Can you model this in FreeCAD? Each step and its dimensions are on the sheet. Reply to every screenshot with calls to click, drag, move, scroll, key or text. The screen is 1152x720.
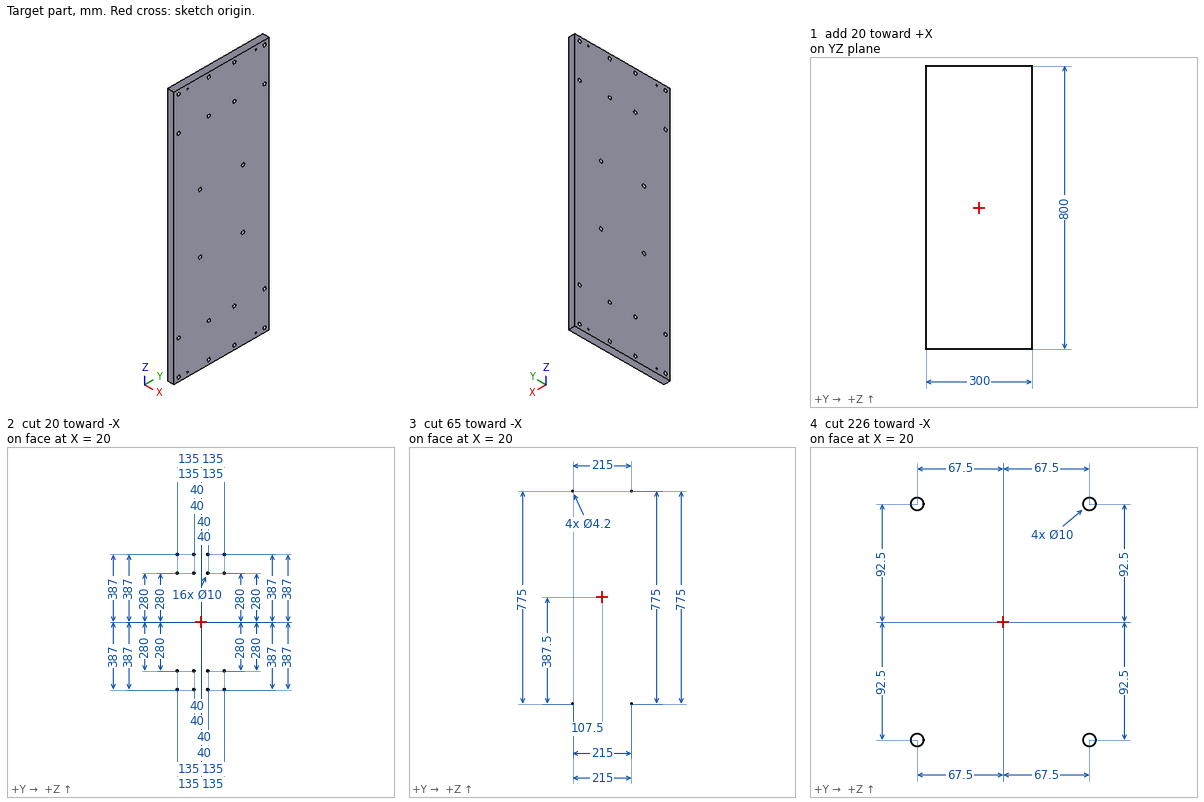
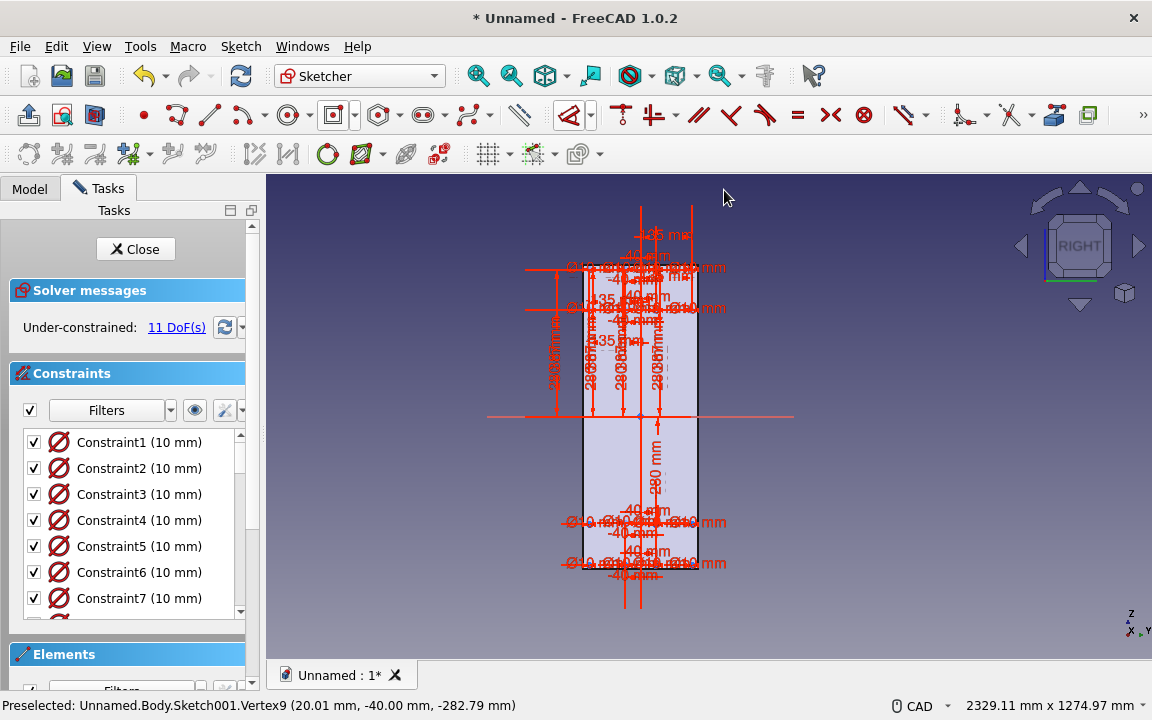
click(589, 524)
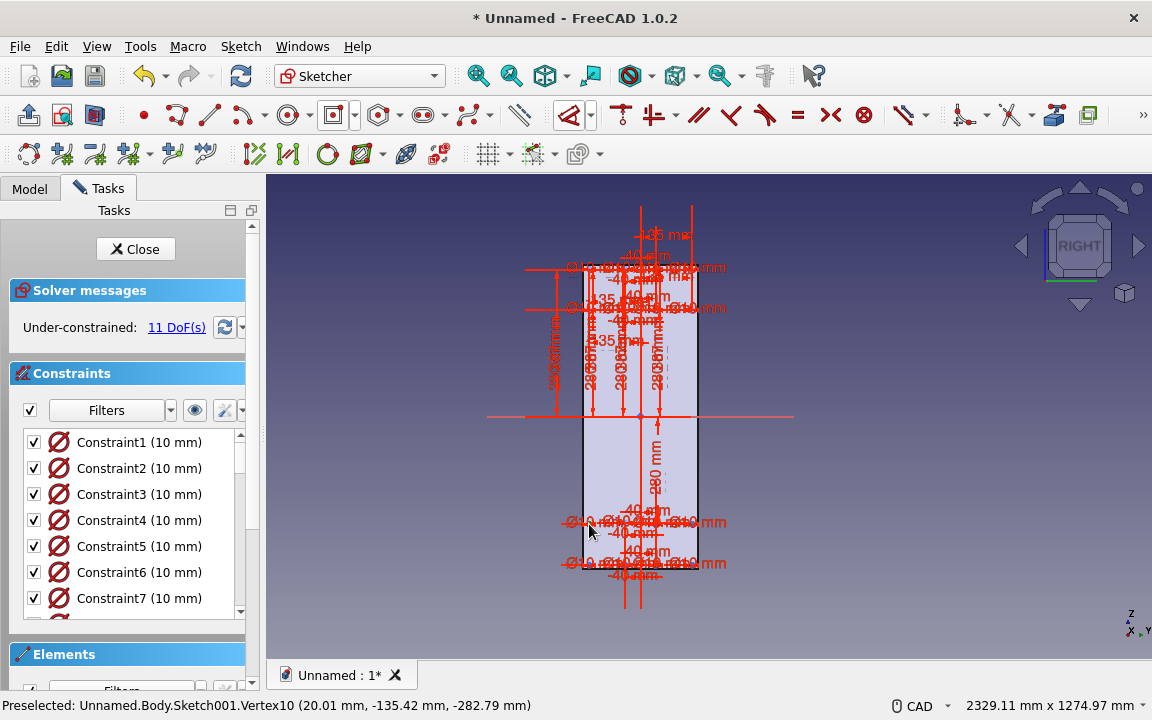
key(l)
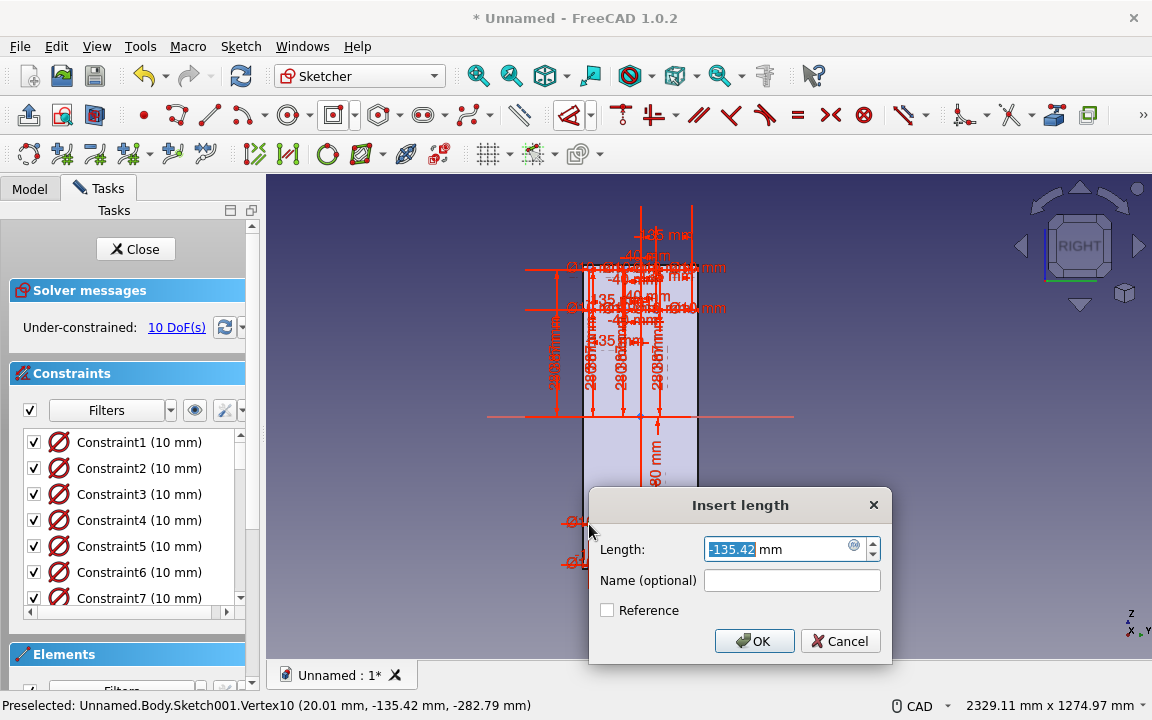
text(-135)
key(Return)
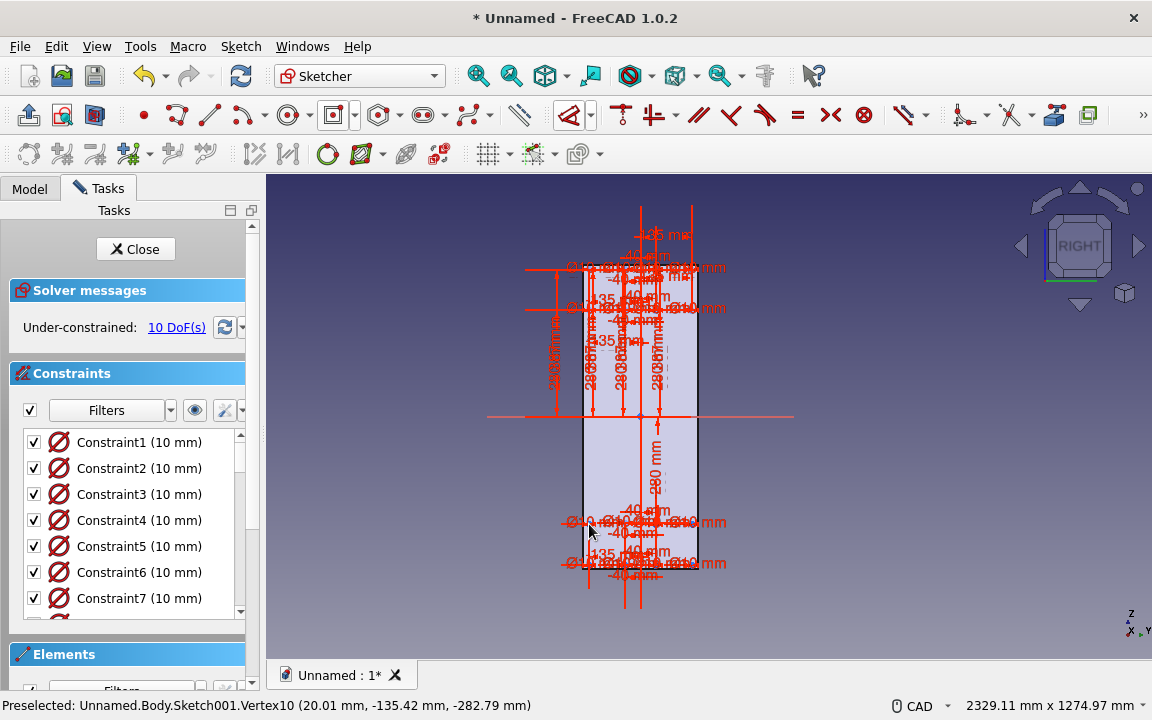
click(589, 524)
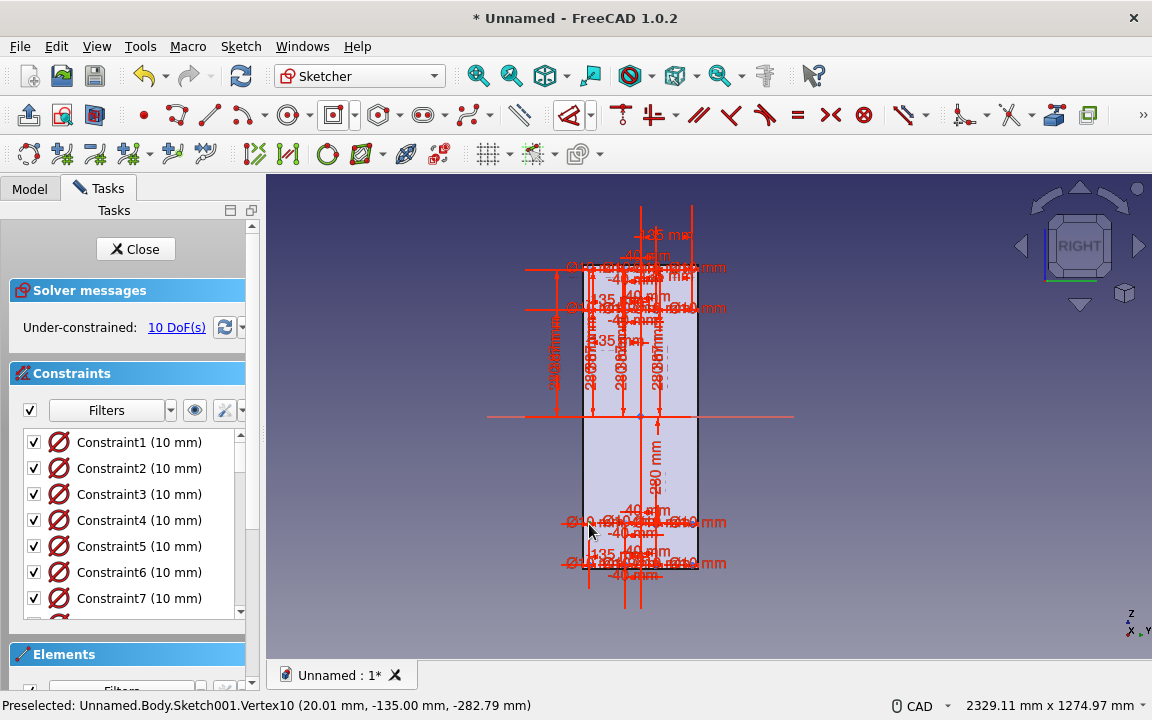
key(i)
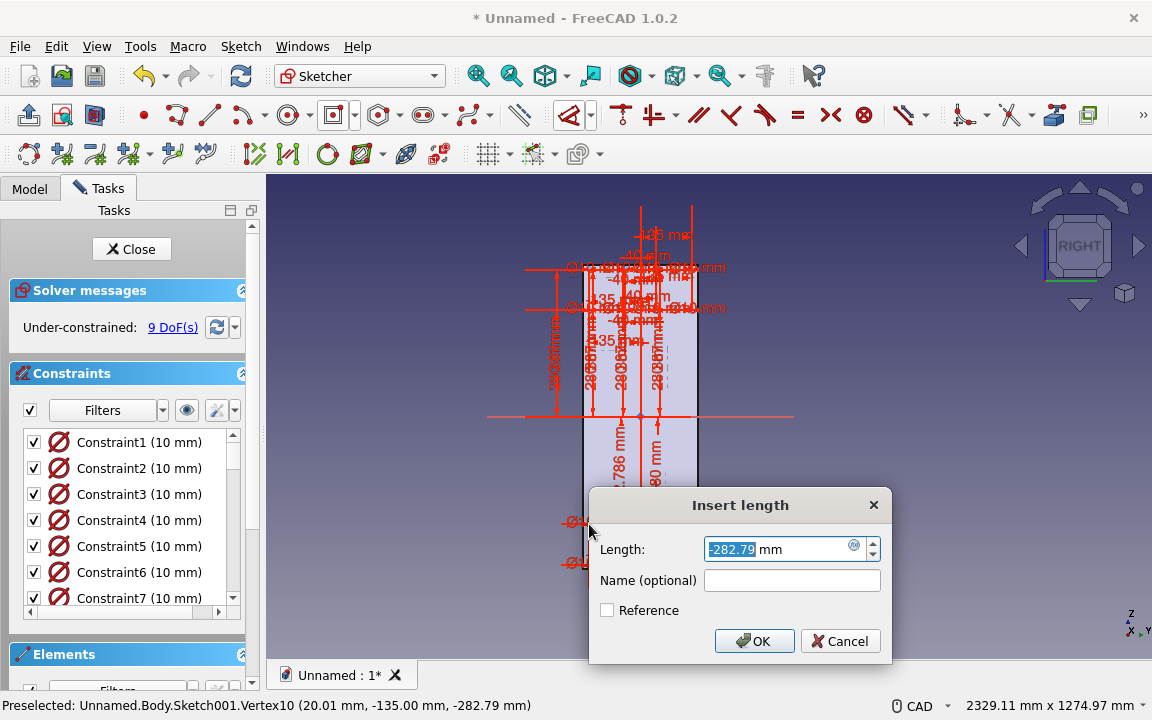
text(-280)
key(Return)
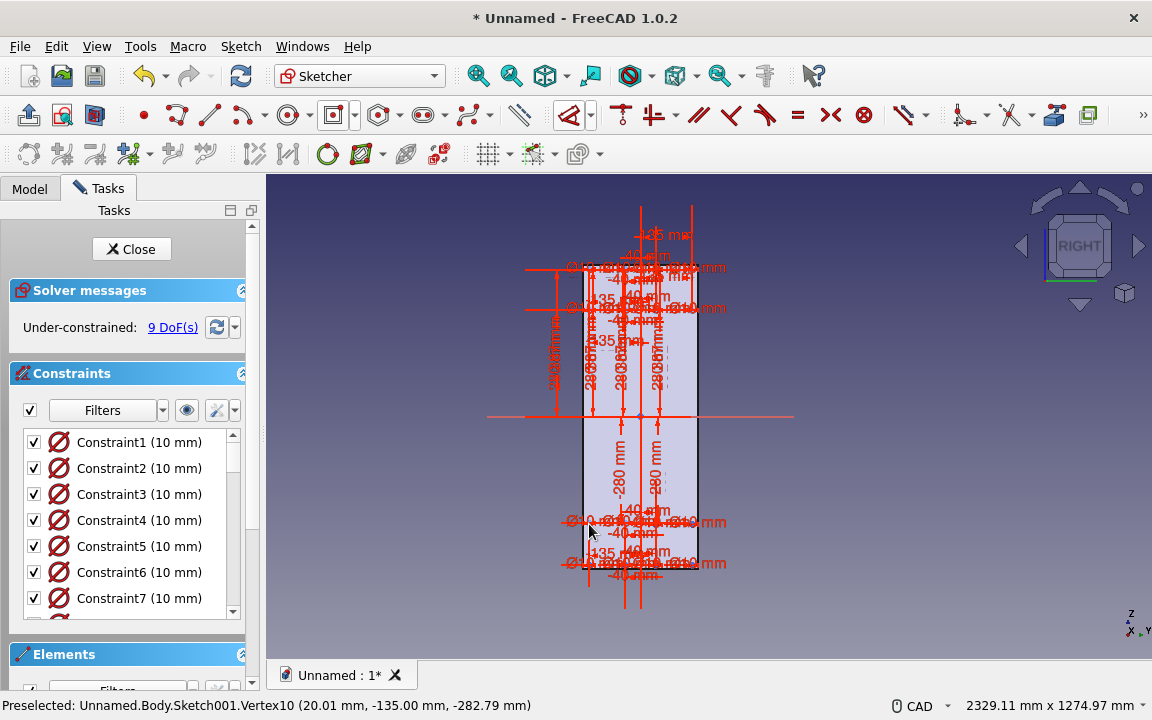
click(589, 565)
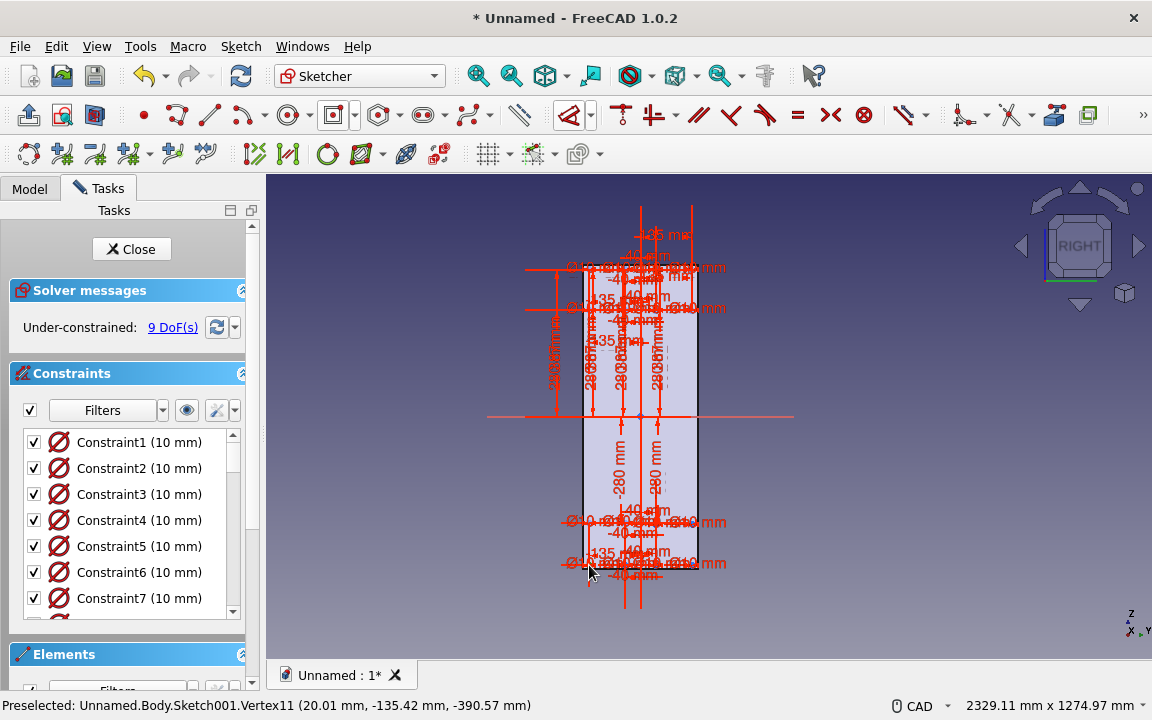
key(l)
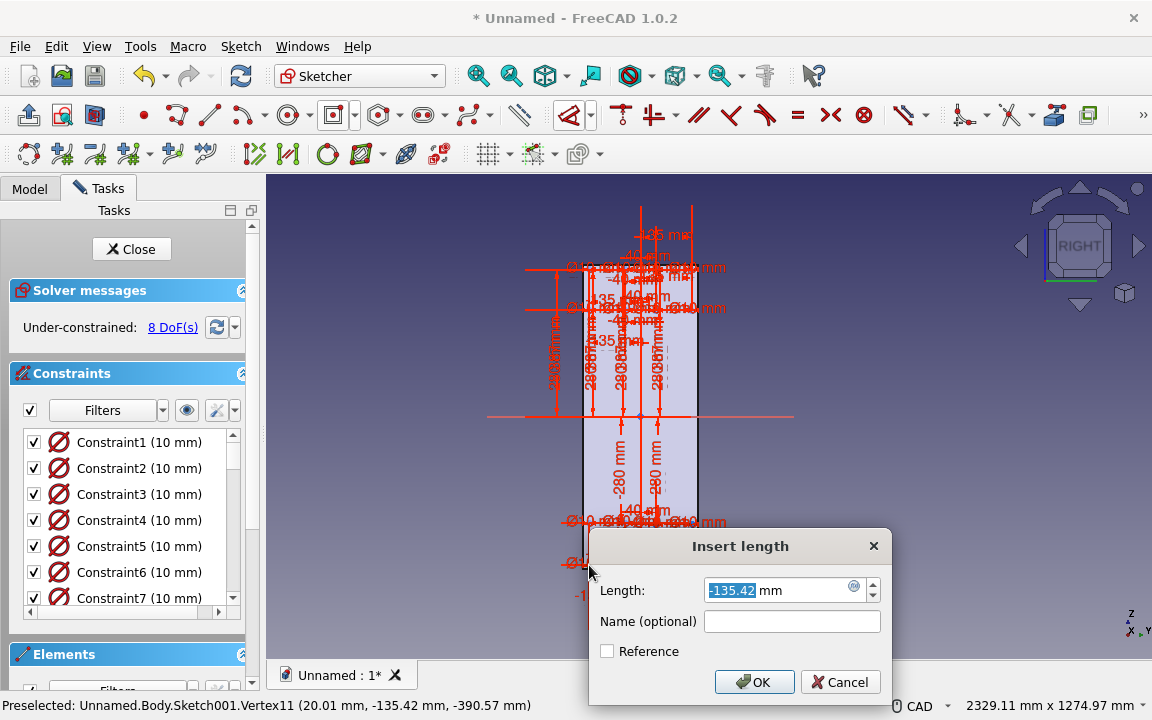
text(-135)
key(Return)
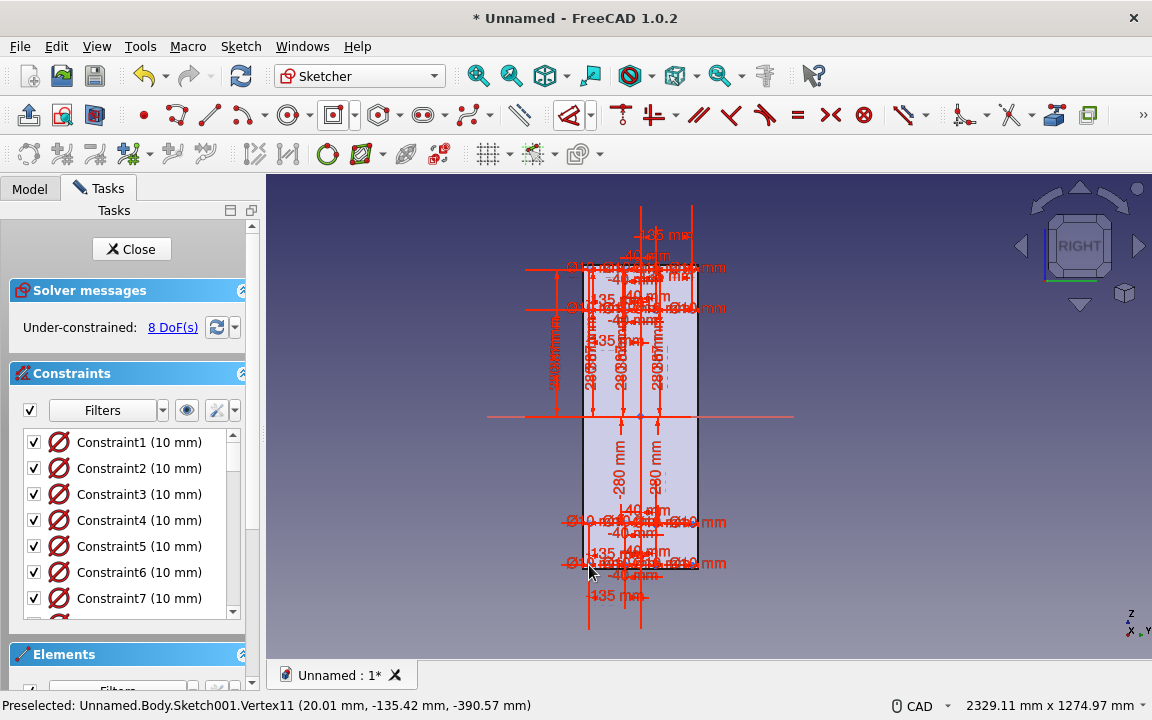
click(589, 565)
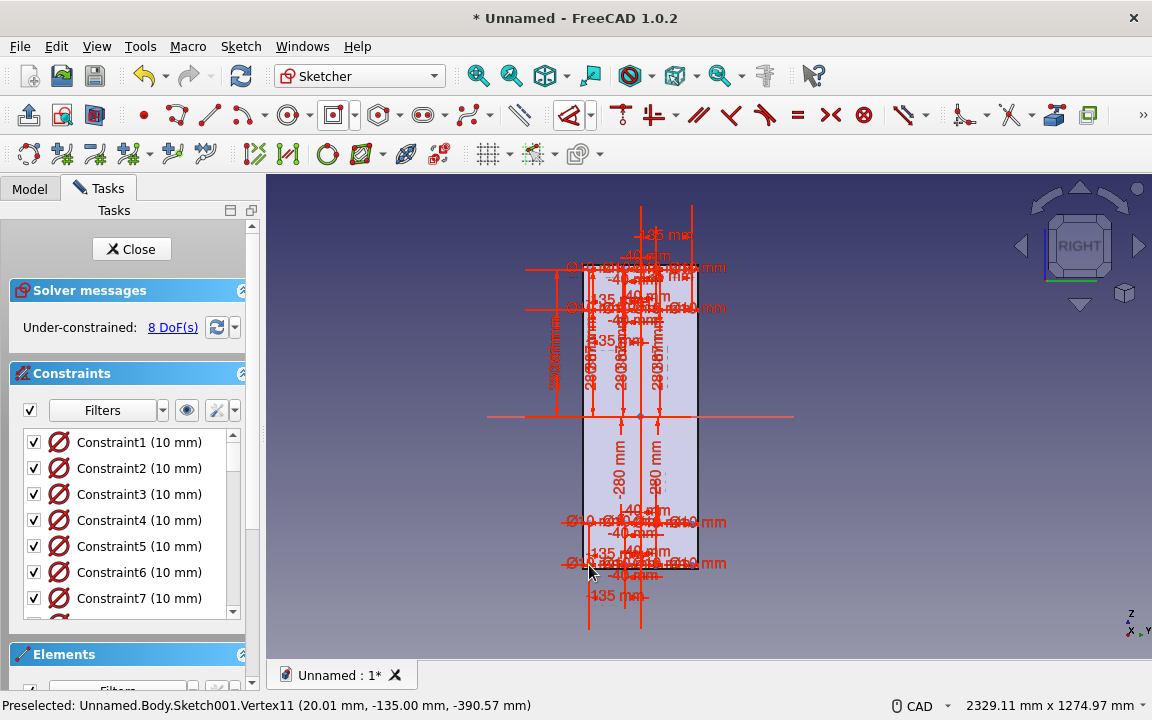
key(i)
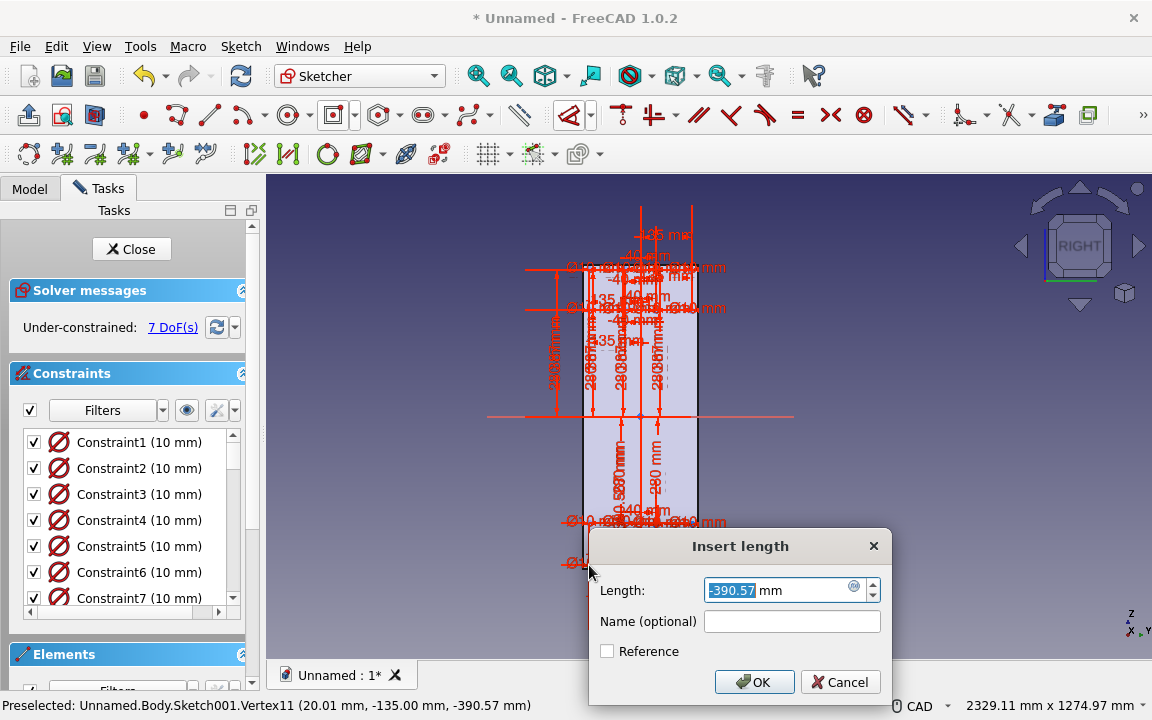
text(-387)
key(Return)